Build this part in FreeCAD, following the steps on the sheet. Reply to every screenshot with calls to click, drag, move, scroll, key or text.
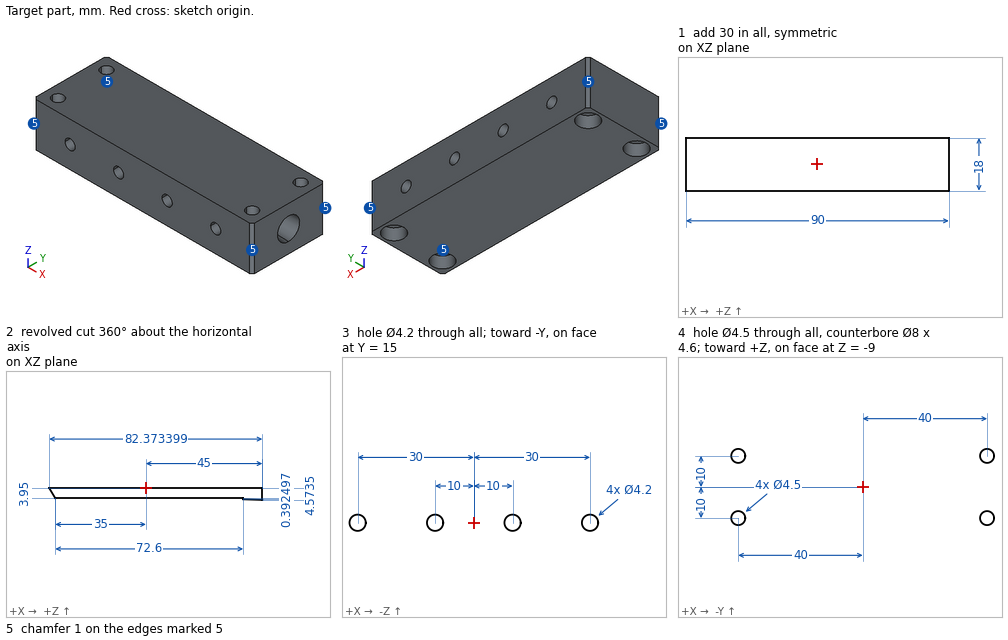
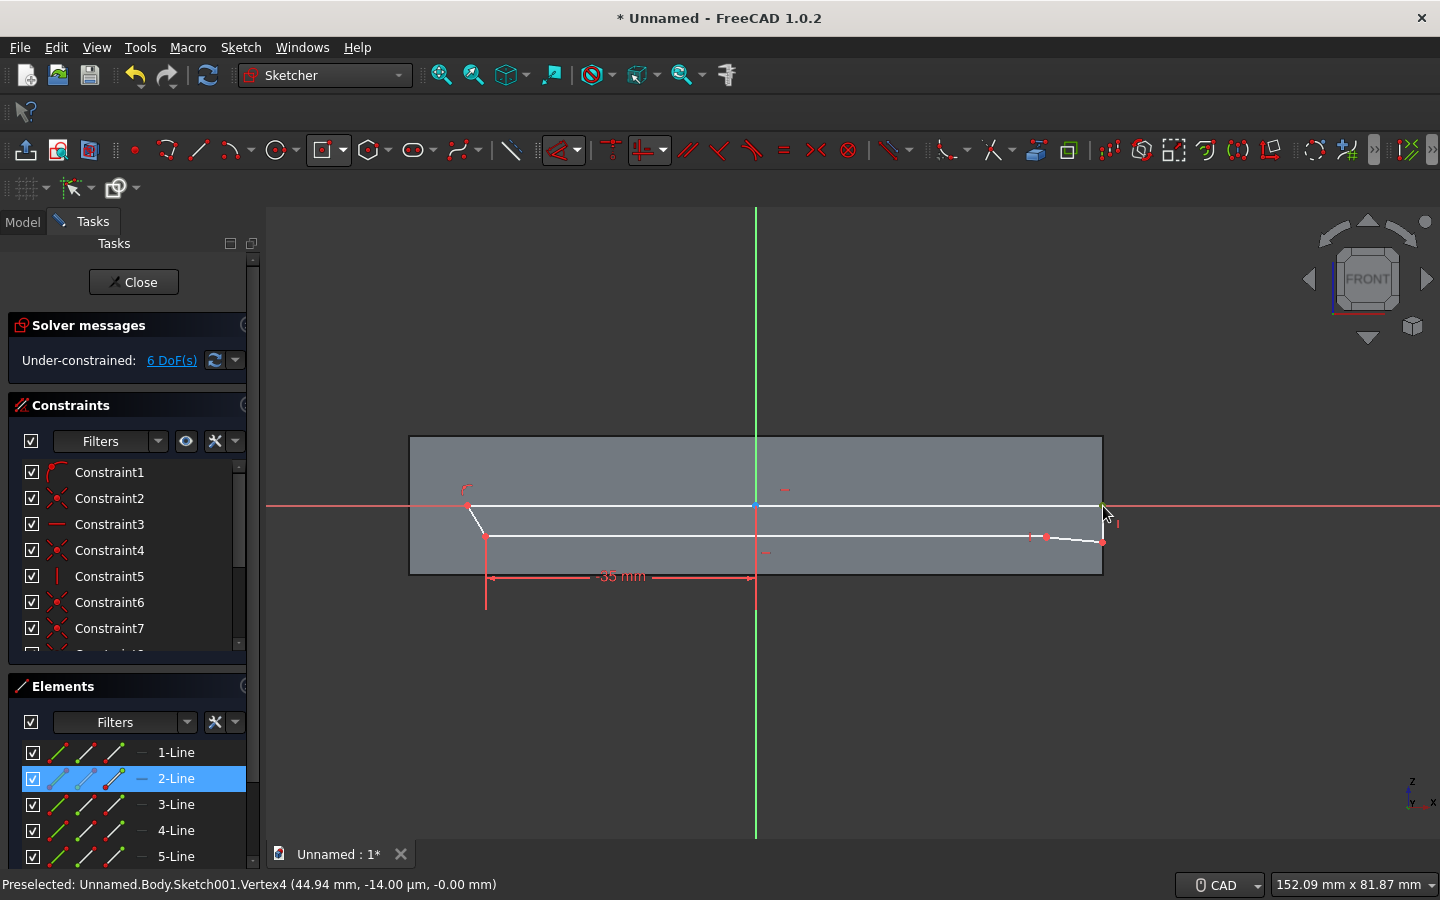
click(580, 150)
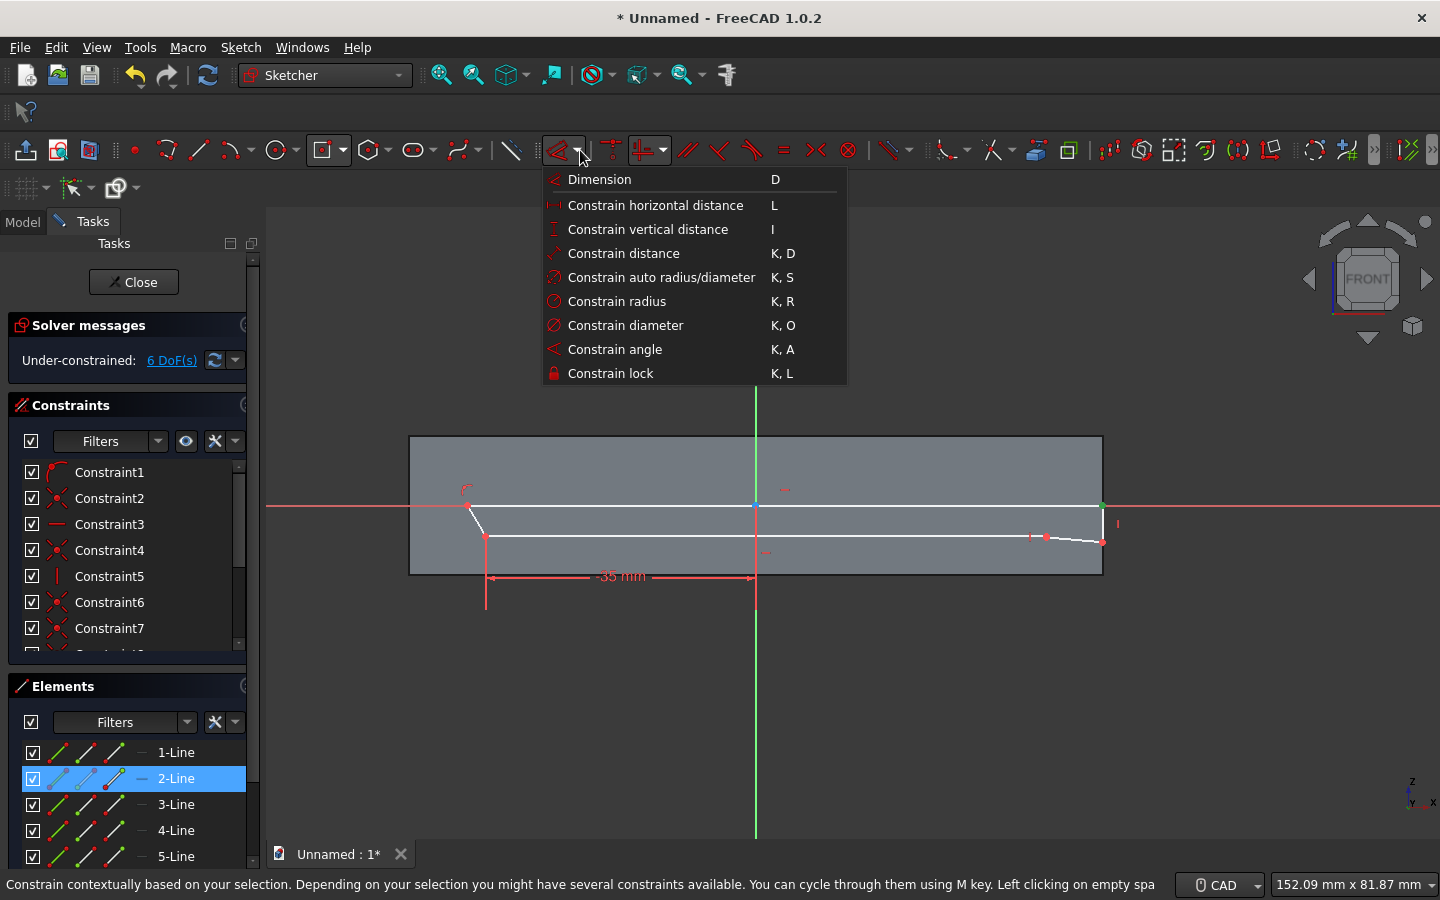
click(695, 205)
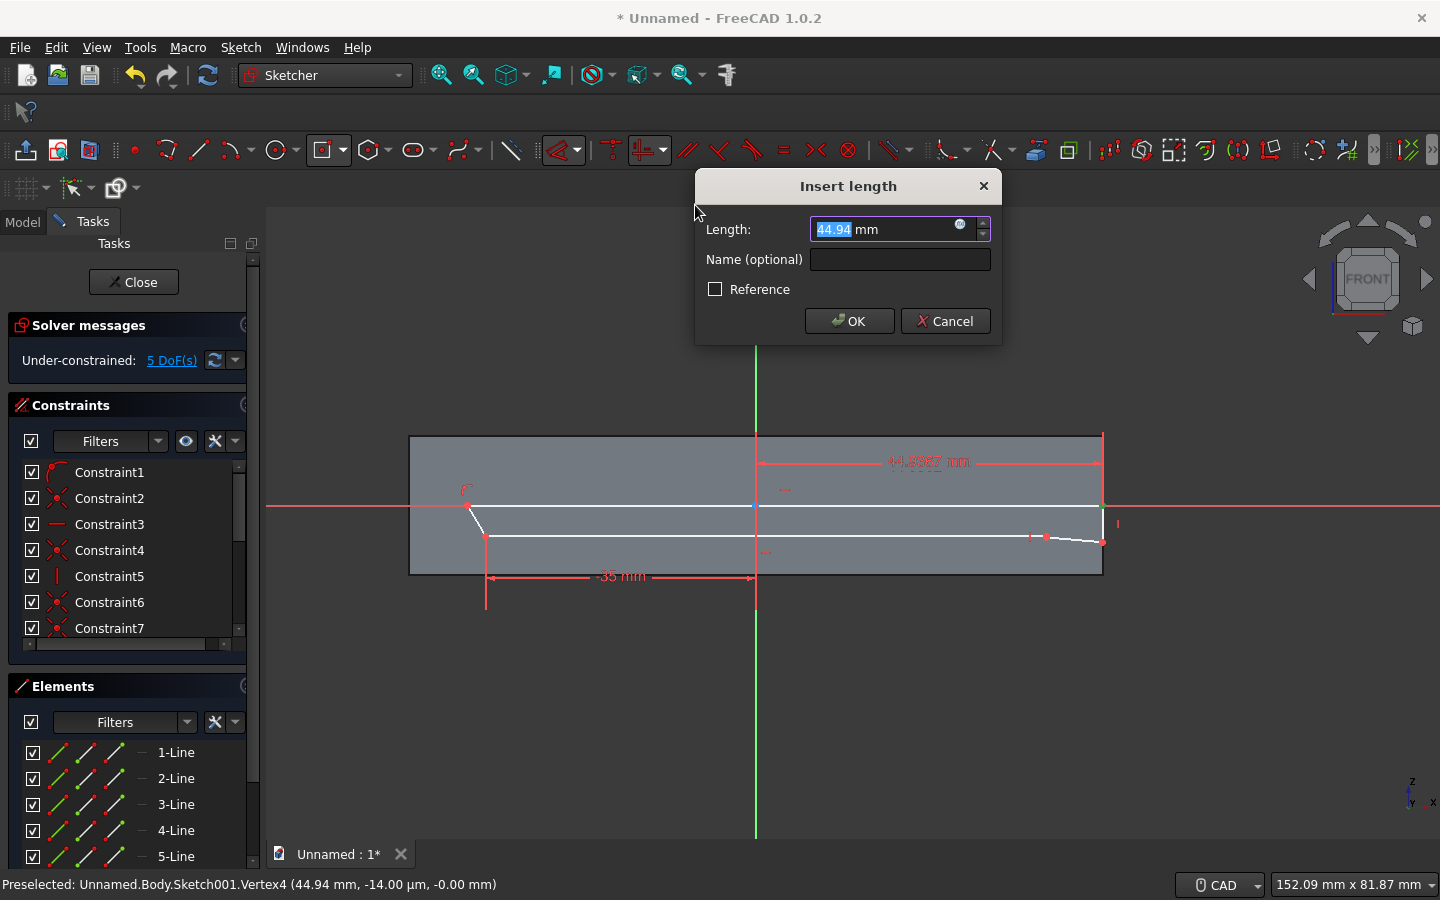
text(45)
key(Return)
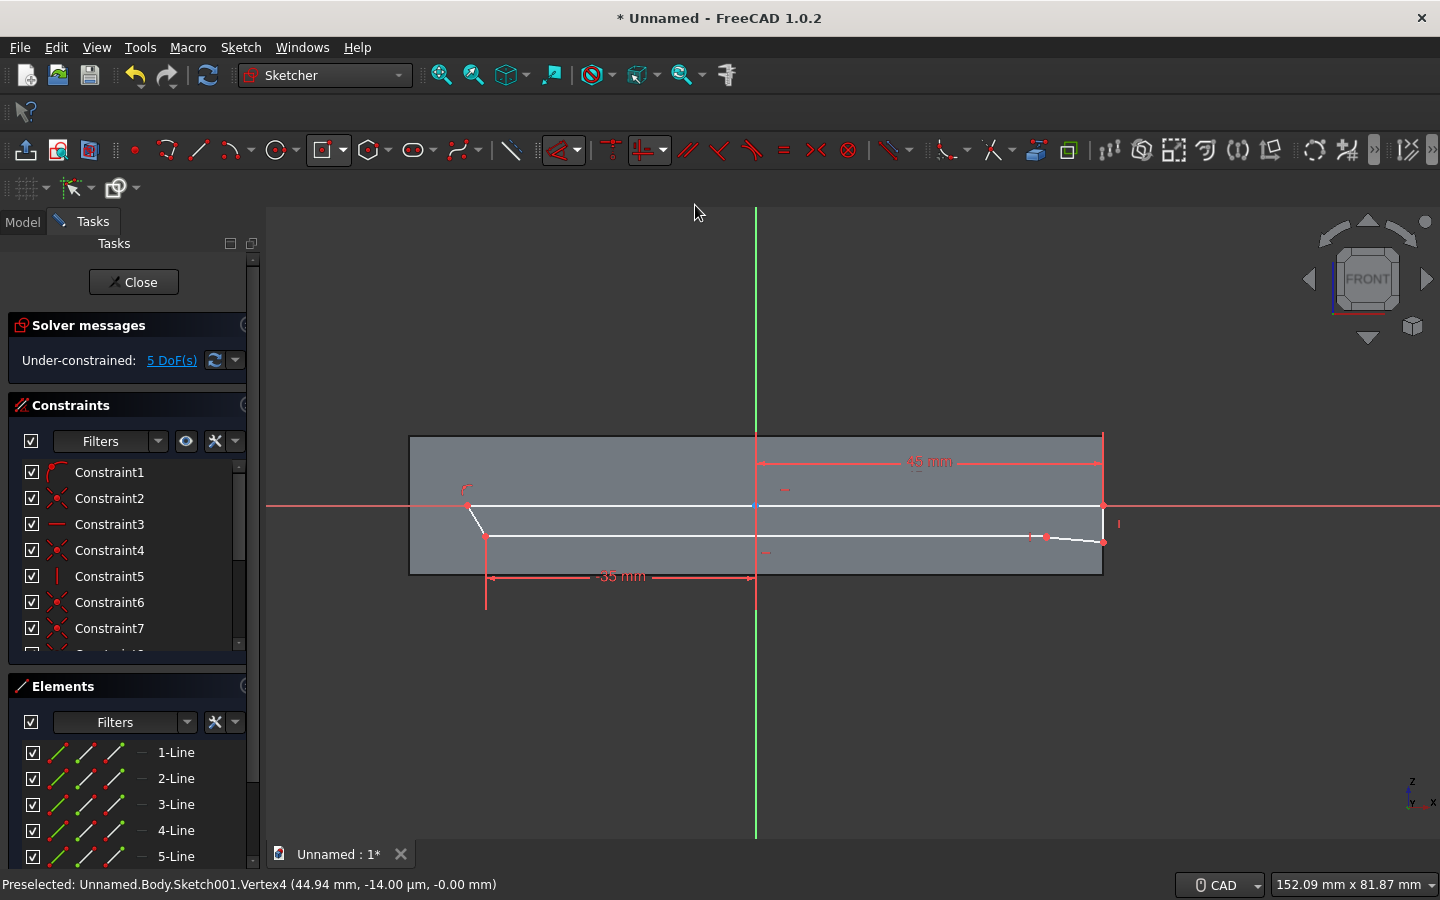
click(878, 536)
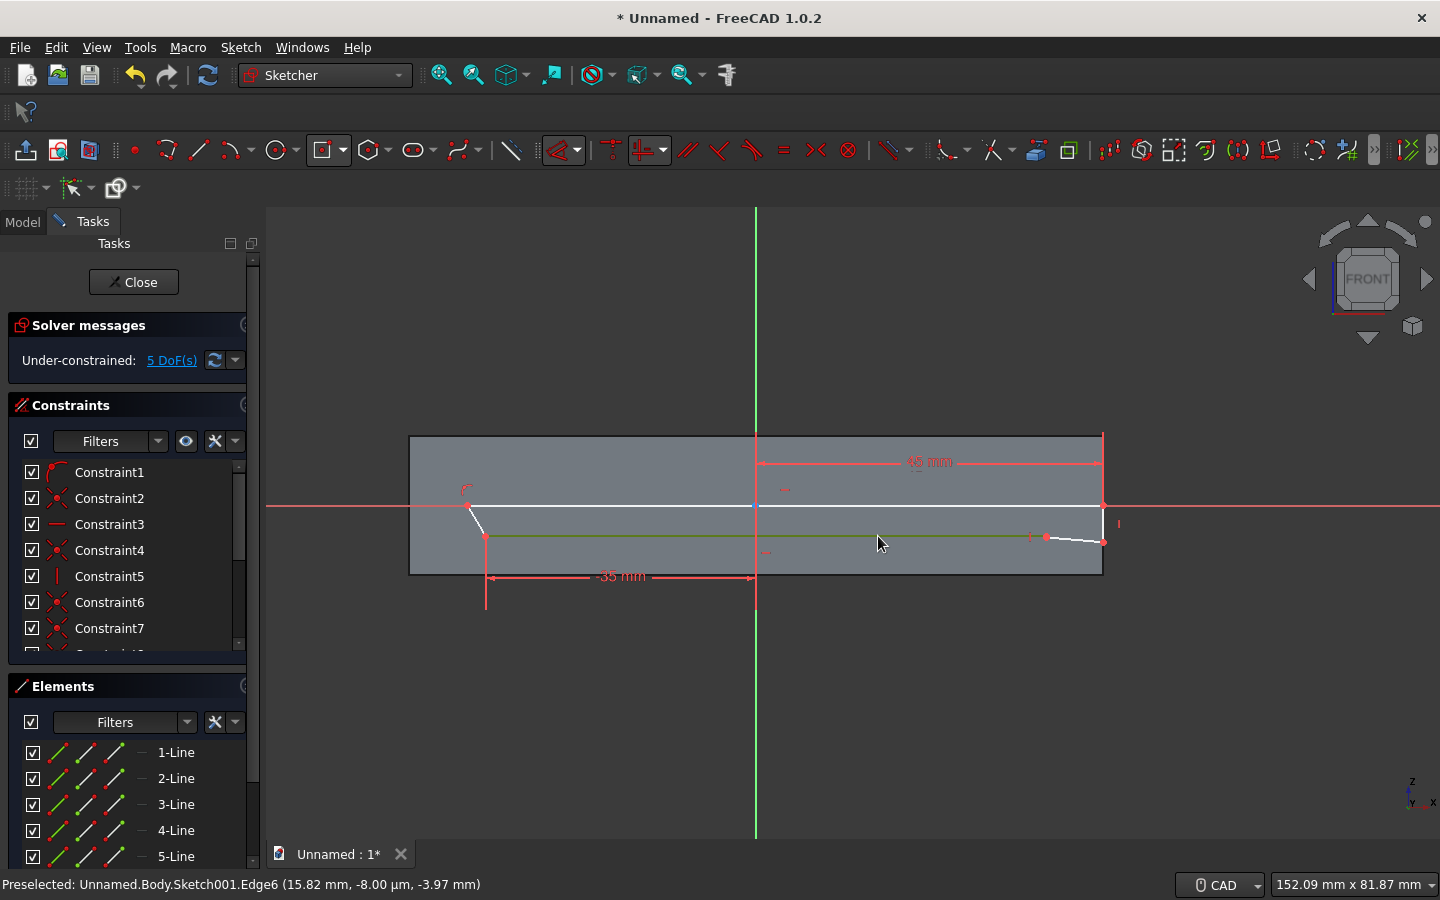
click(580, 150)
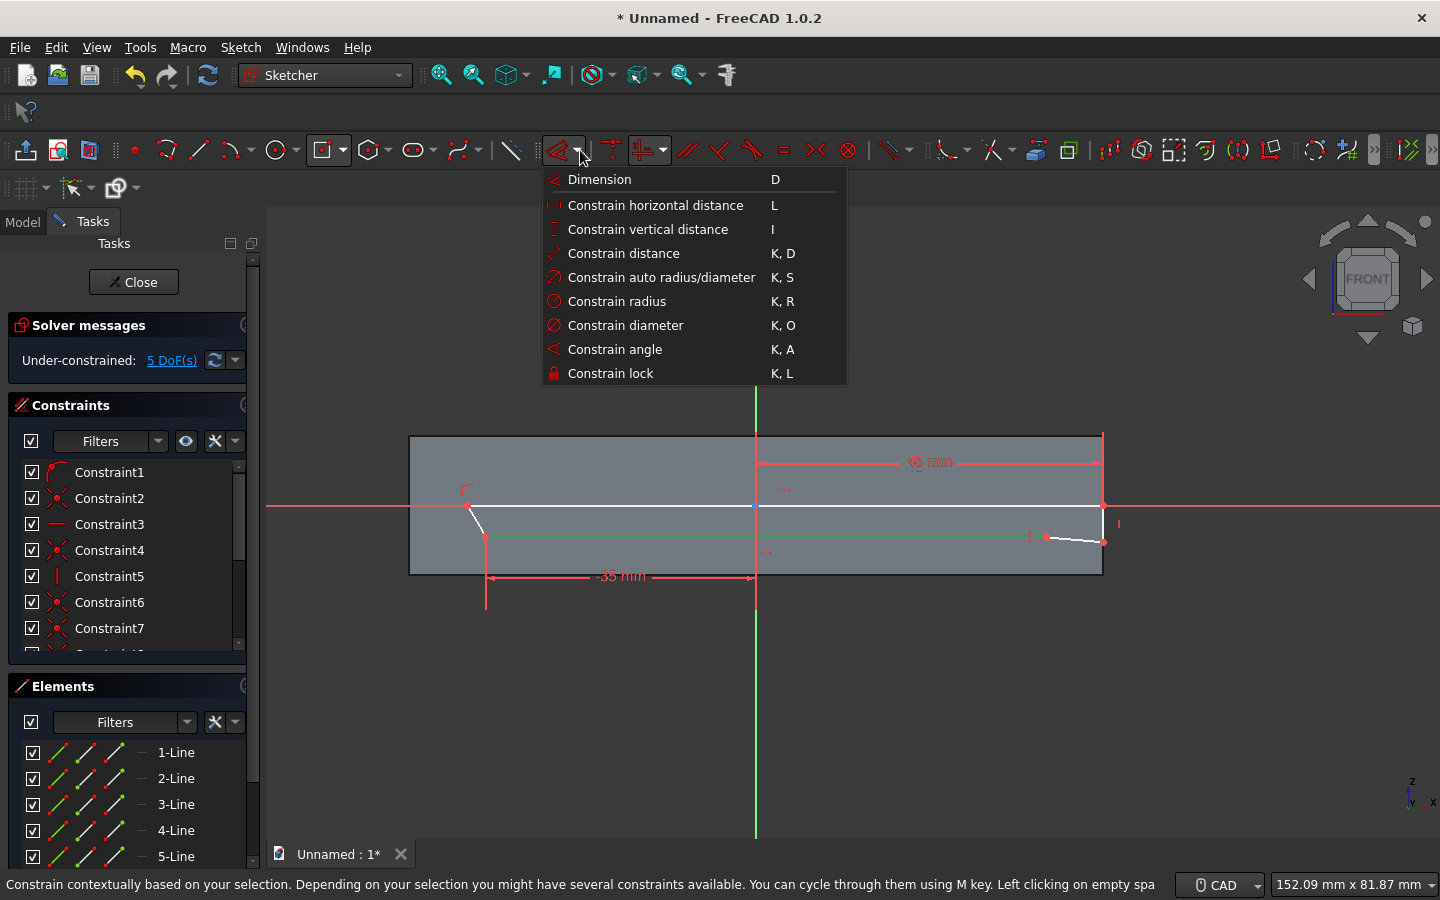
click(695, 205)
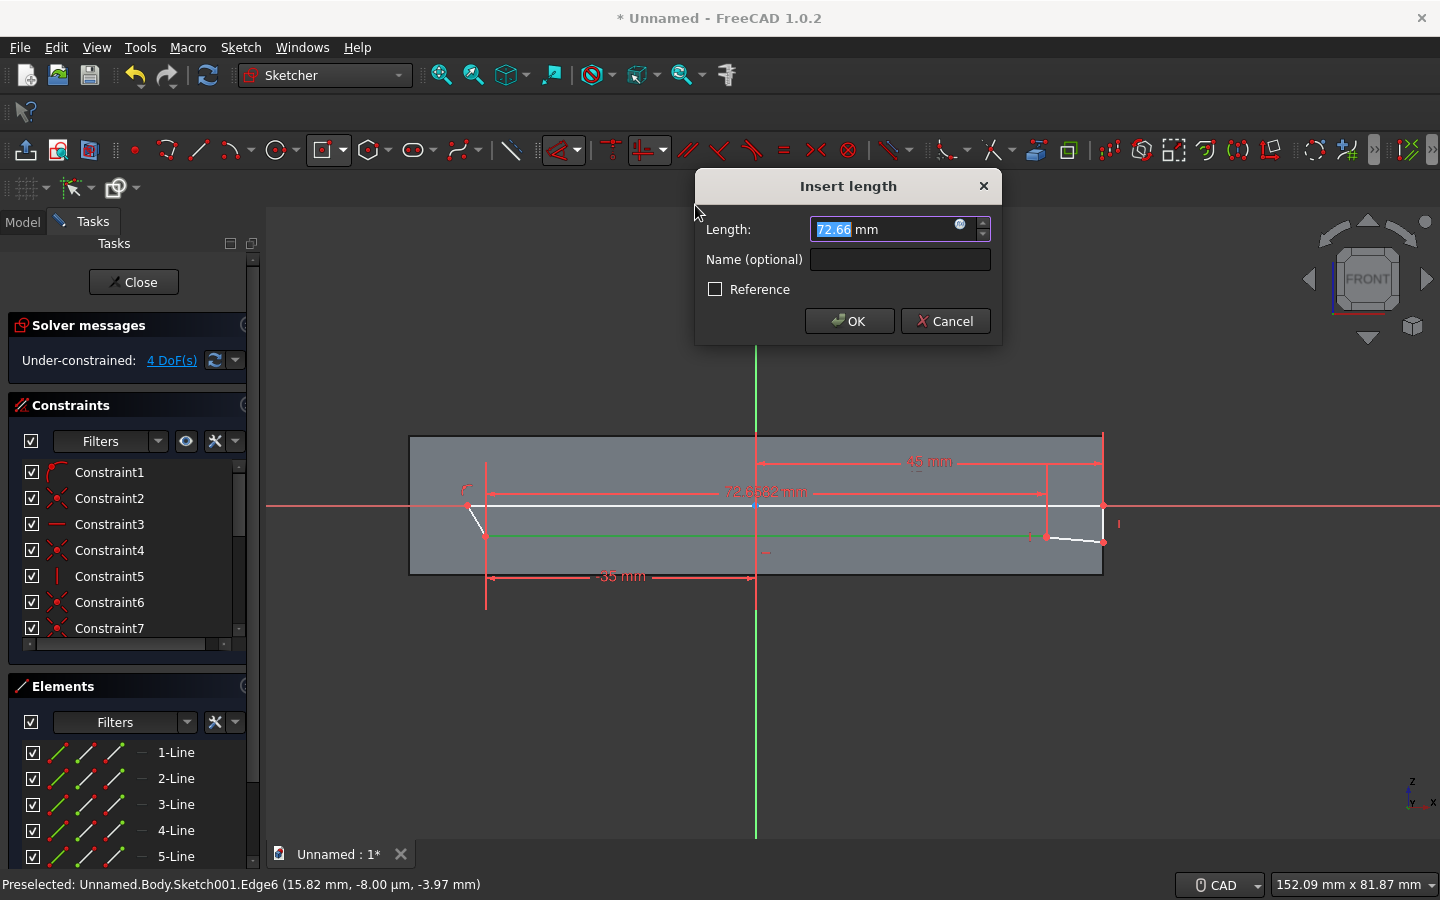
text(72.6)
key(Return)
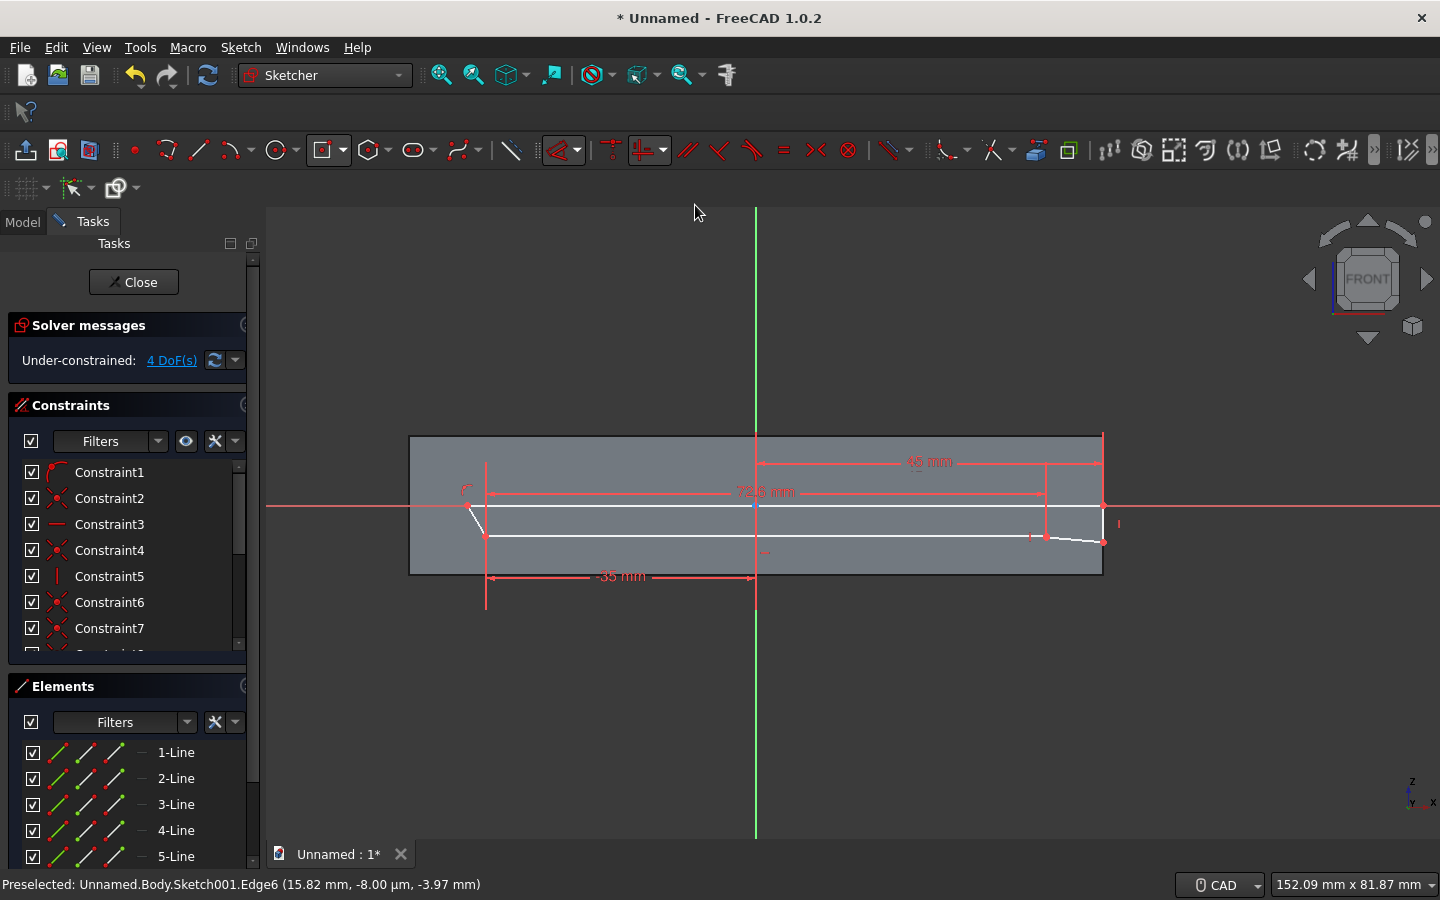
scroll(486, 536, up, 2)